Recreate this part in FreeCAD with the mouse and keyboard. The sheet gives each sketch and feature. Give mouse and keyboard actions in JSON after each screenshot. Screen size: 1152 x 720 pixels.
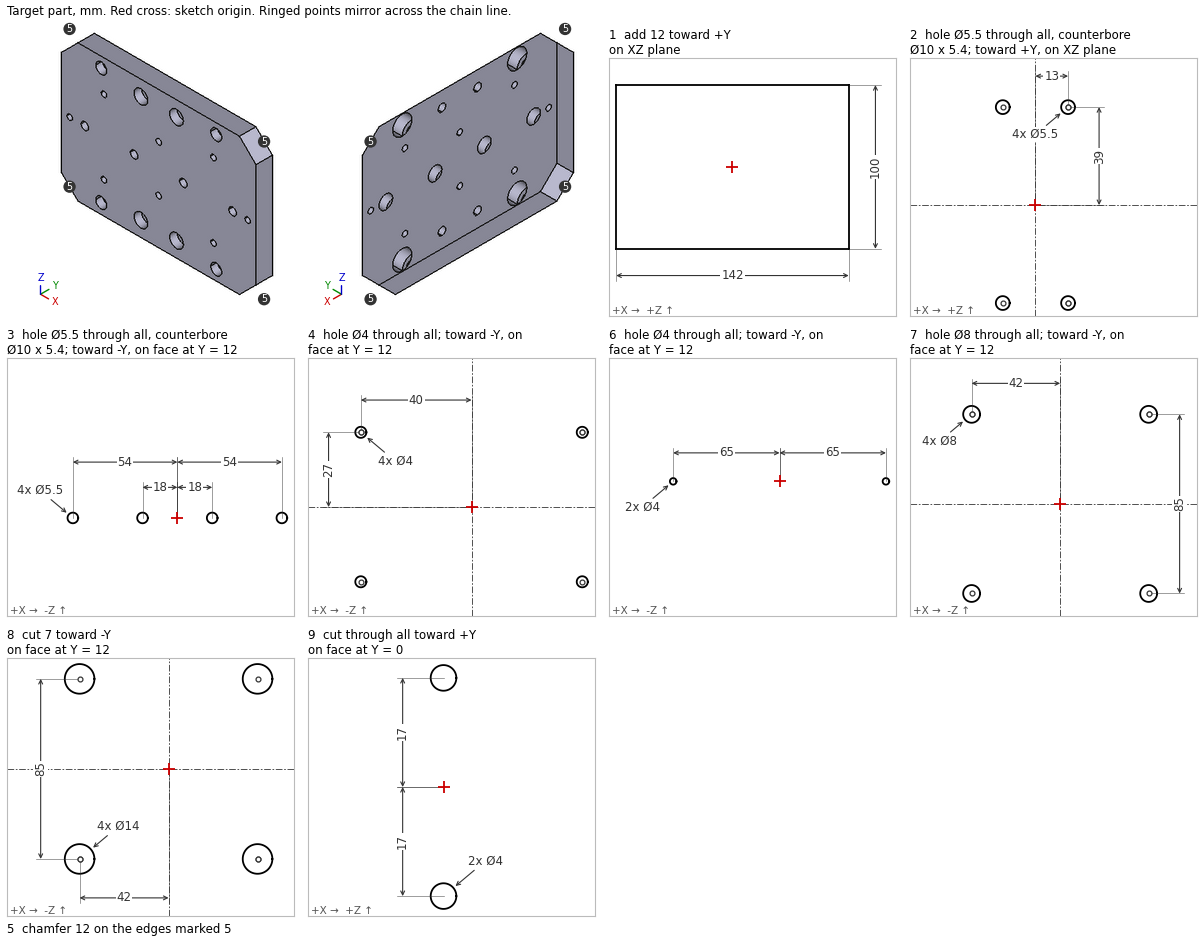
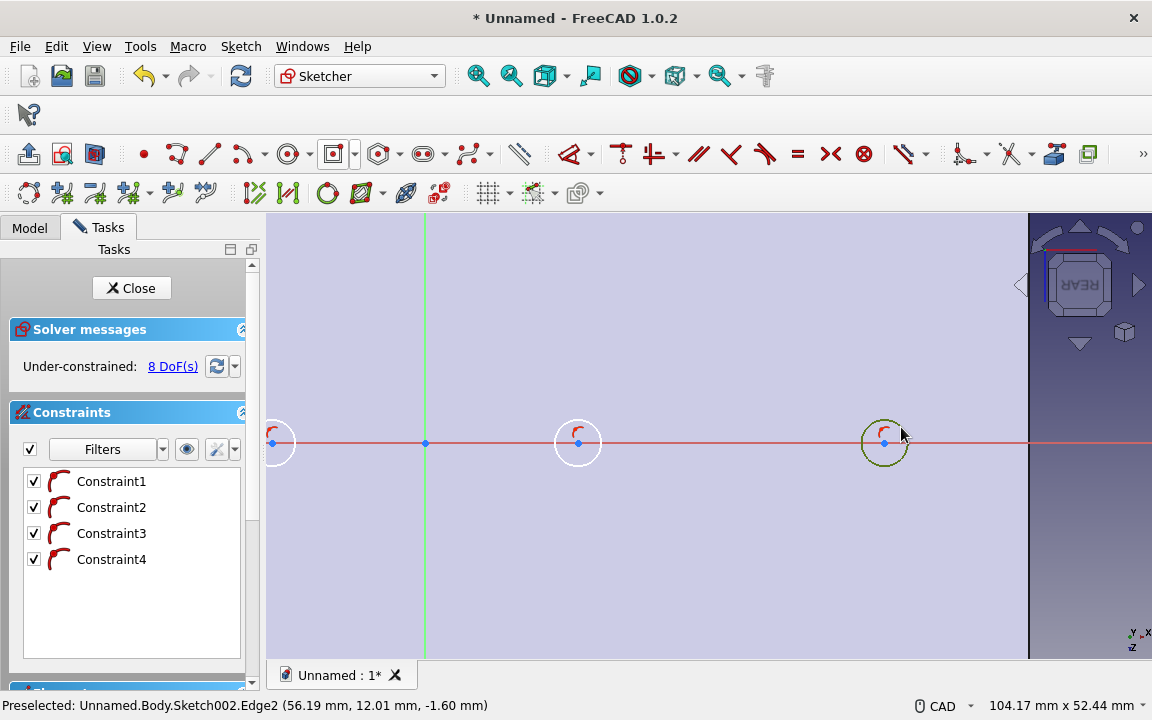
{"action": "left_click", "coordinate": [295, 444]}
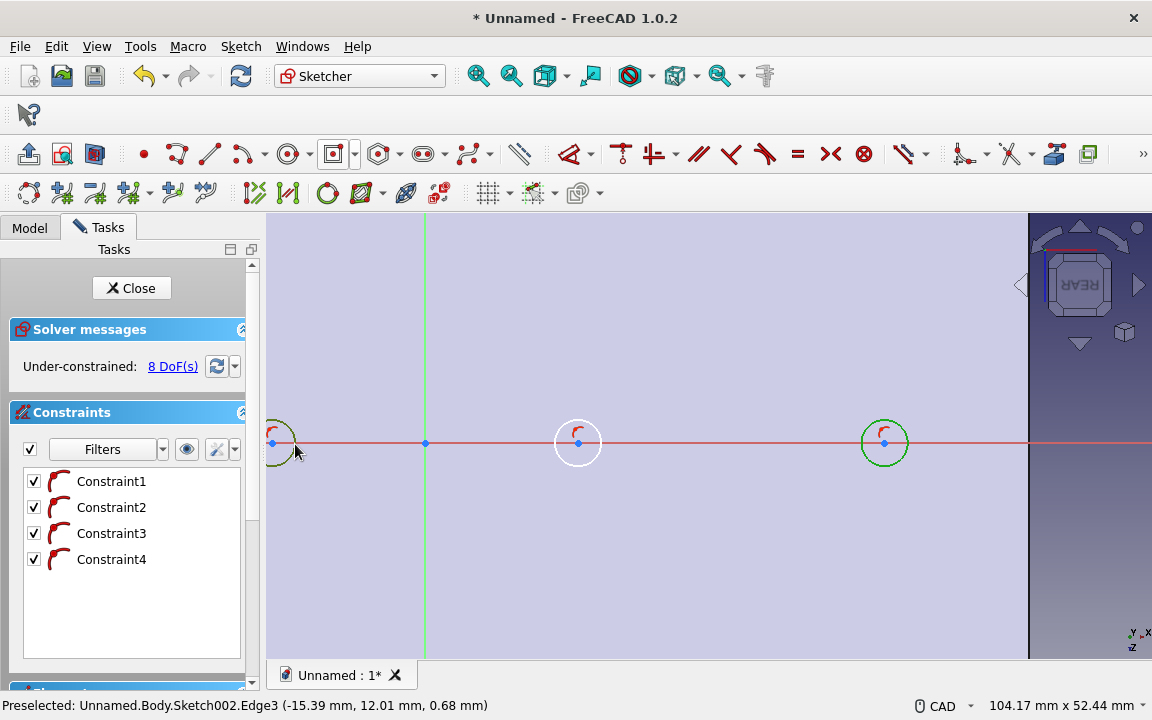
{"action": "left_click", "coordinate": [594, 427]}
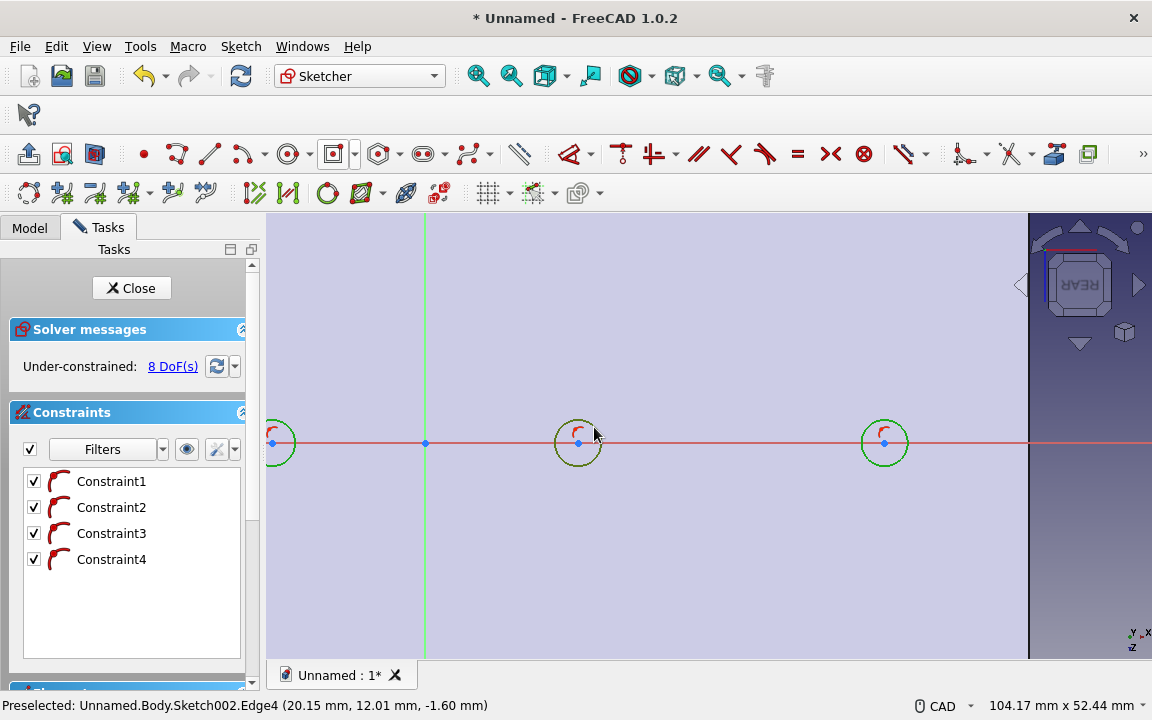
{"action": "left_click", "coordinate": [798, 154]}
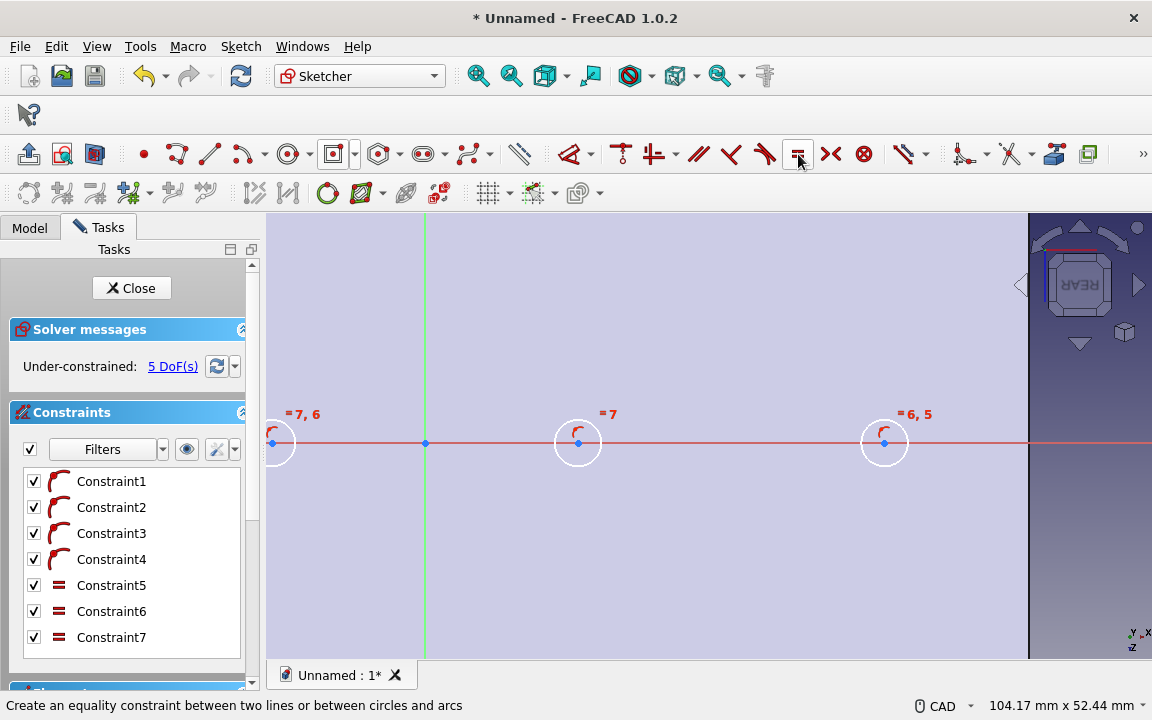
{"action": "left_click", "coordinate": [568, 154]}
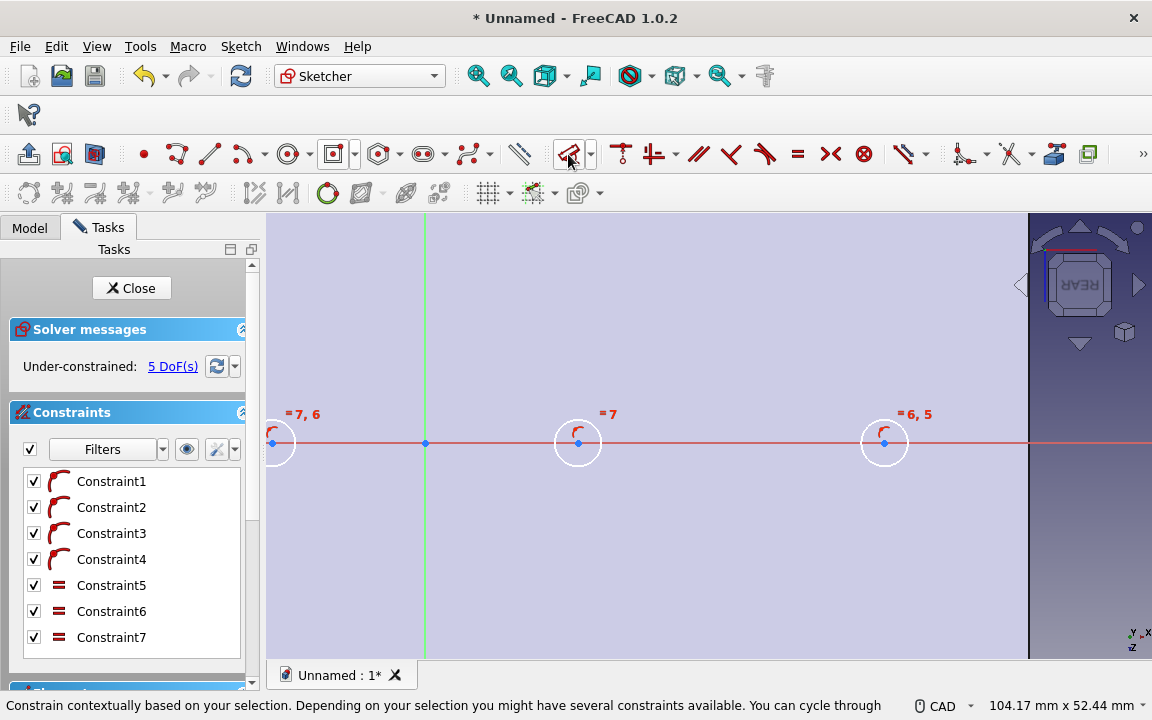
{"action": "scroll", "coordinate": [902, 427], "scroll_direction": "down", "scroll_amount": 3}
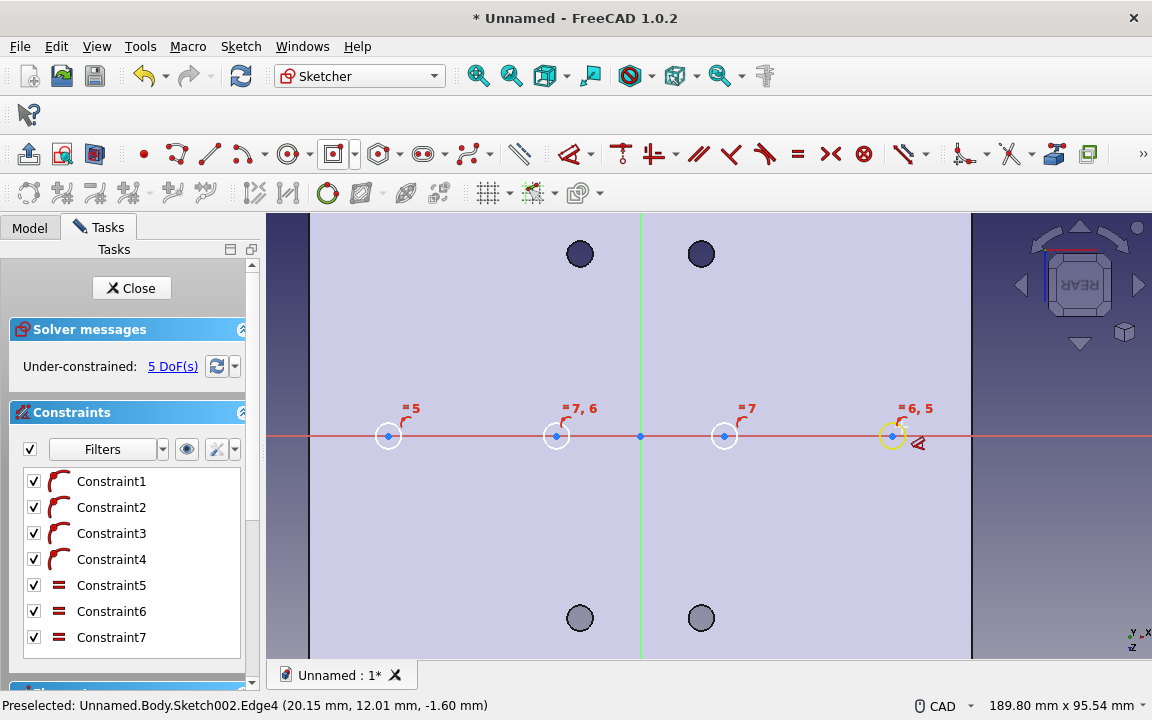
{"action": "scroll", "coordinate": [398, 427], "scroll_direction": "up", "scroll_amount": 3}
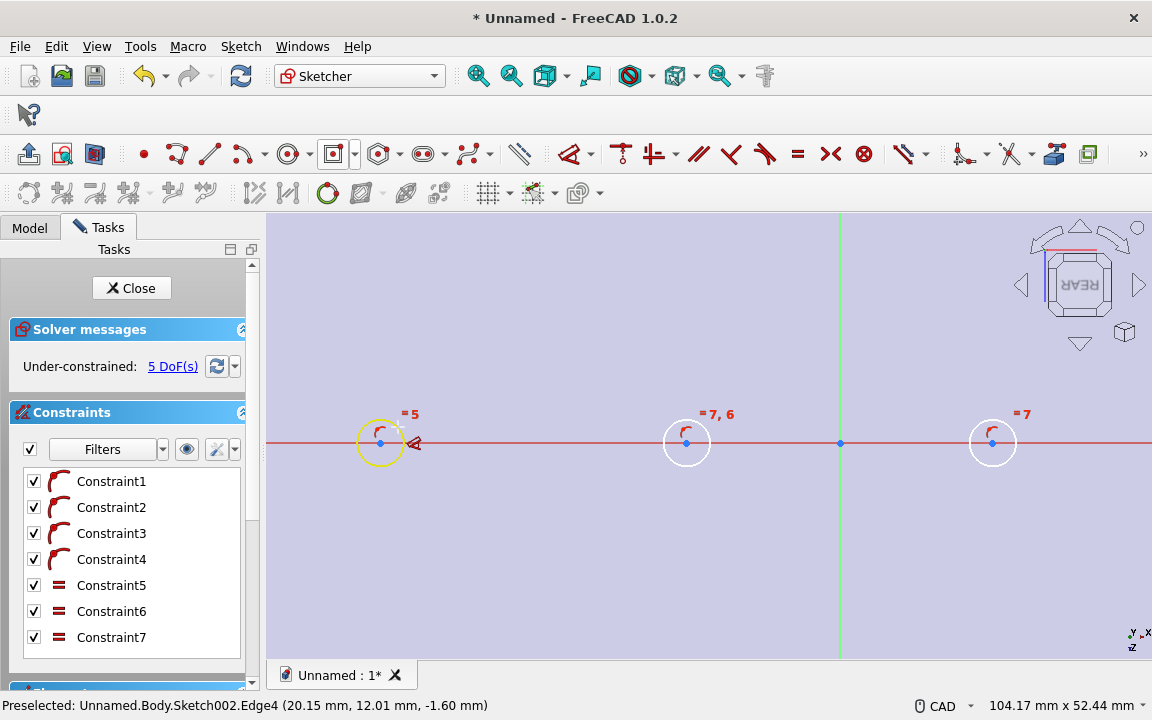
{"action": "left_click", "coordinate": [397, 427]}
{"action": "left_click", "coordinate": [420, 405]}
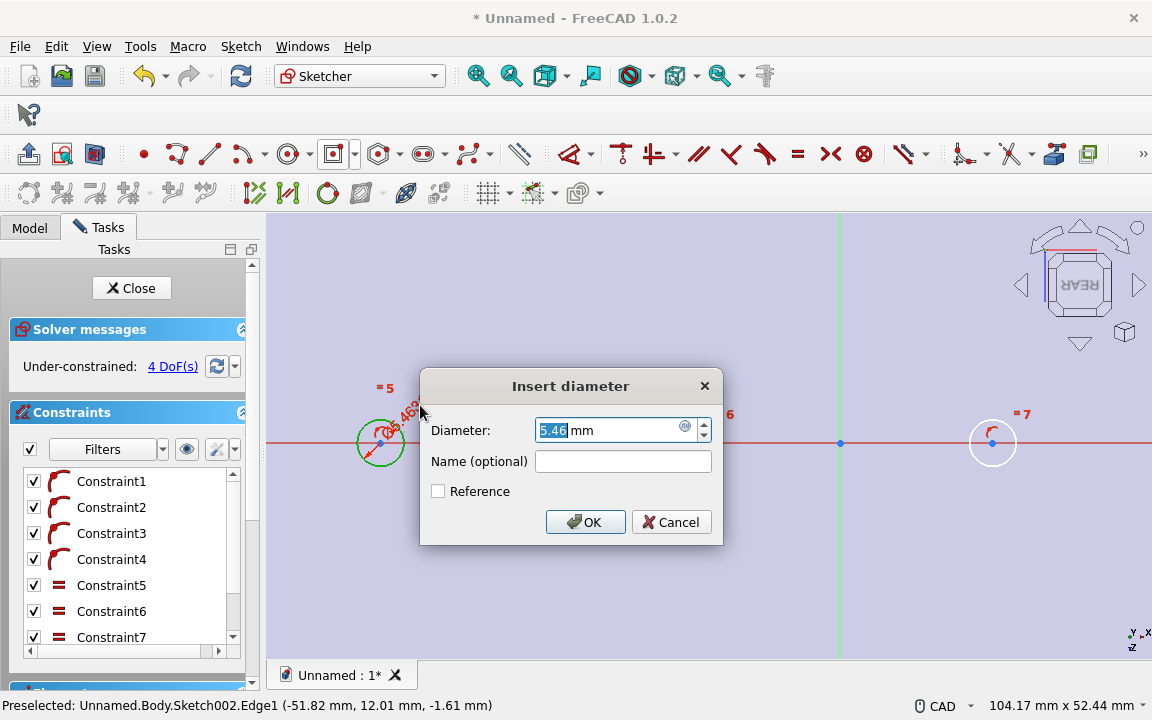
{"action": "type", "text": "5.5"}
{"action": "key", "text": "Return"}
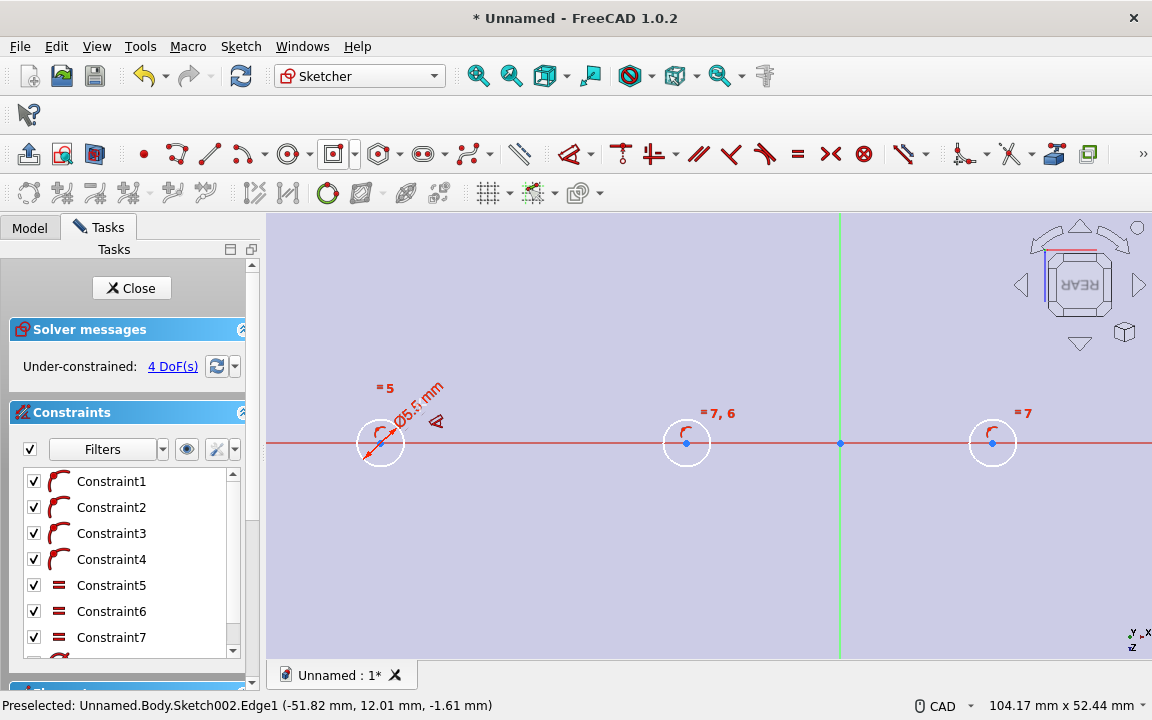
{"action": "left_click", "coordinate": [381, 443]}
{"action": "left_click", "coordinate": [610, 477]}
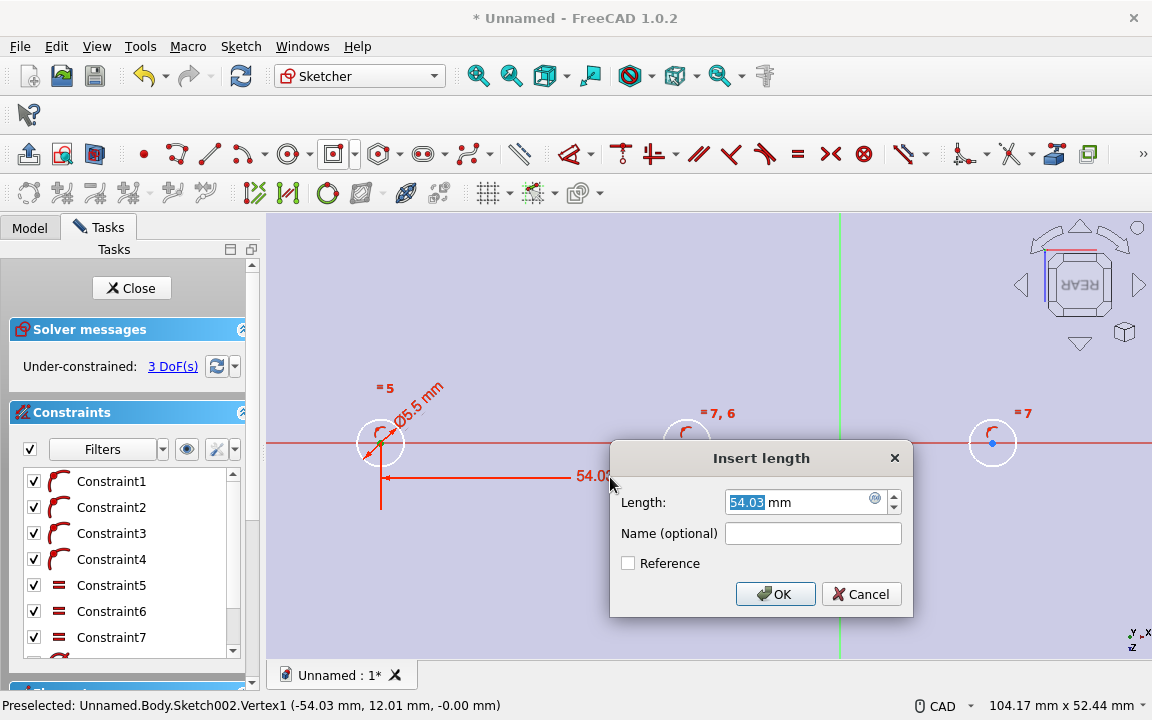
{"action": "type", "text": "54"}
{"action": "key", "text": "Return"}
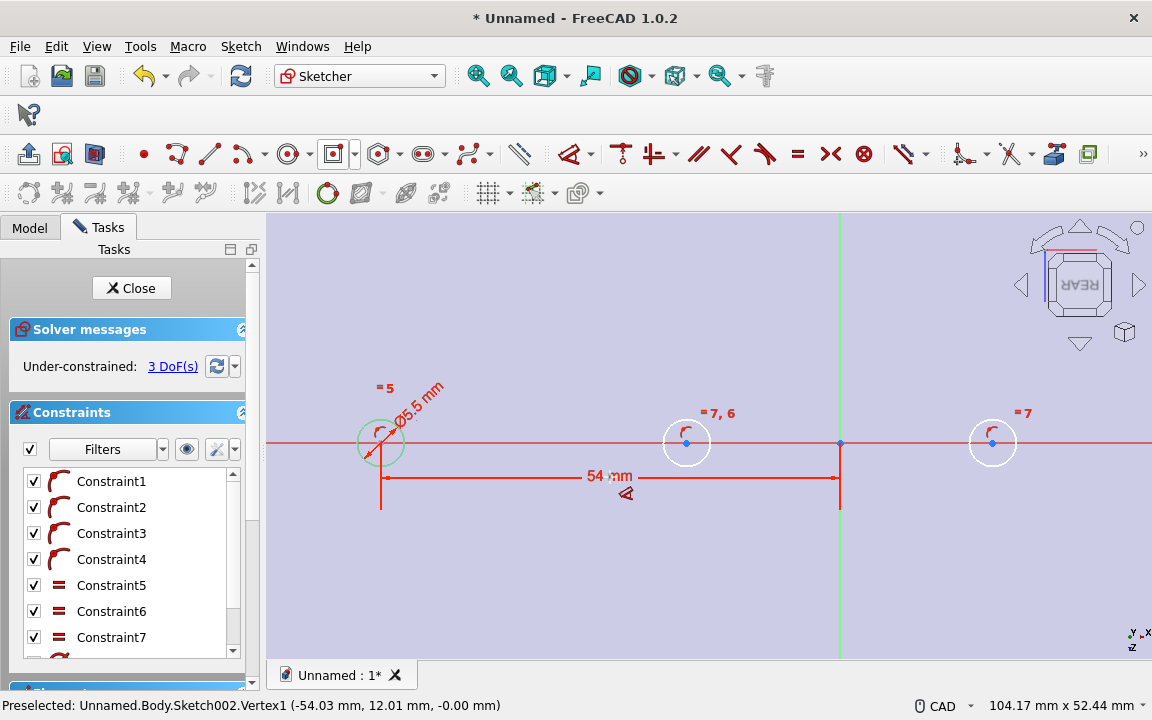
{"action": "scroll", "coordinate": [398, 427], "scroll_direction": "down", "scroll_amount": 3}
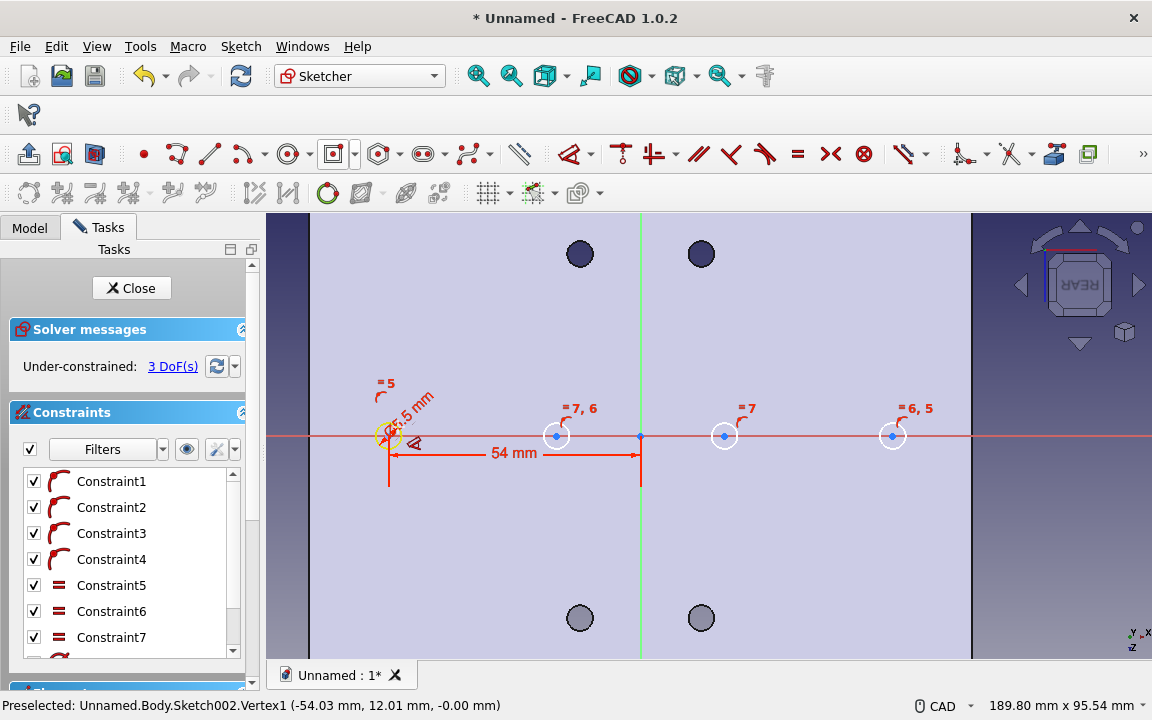
{"action": "left_click", "coordinate": [893, 436]}
{"action": "left_click", "coordinate": [767, 470]}